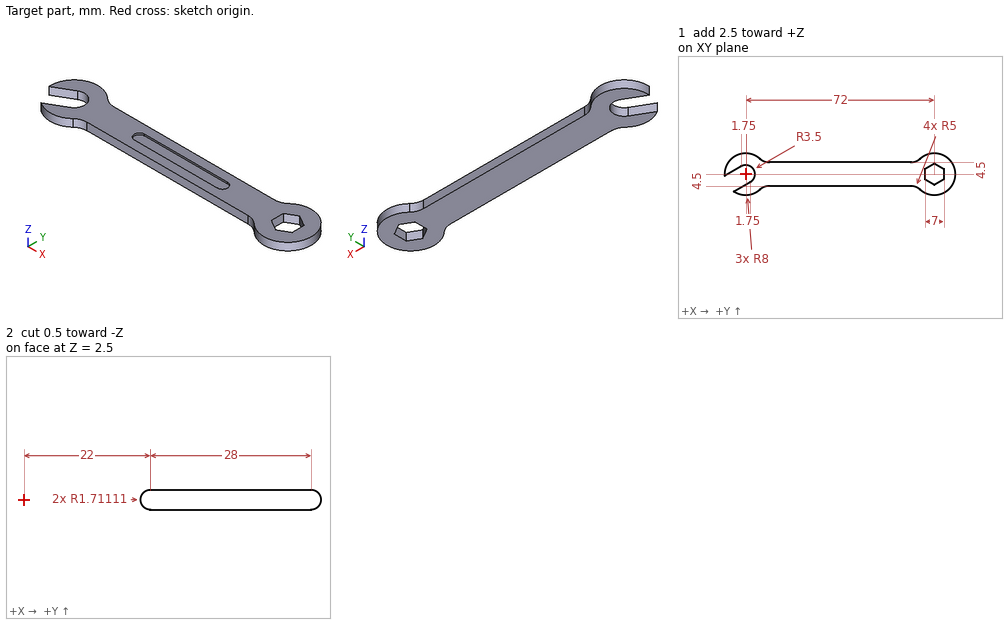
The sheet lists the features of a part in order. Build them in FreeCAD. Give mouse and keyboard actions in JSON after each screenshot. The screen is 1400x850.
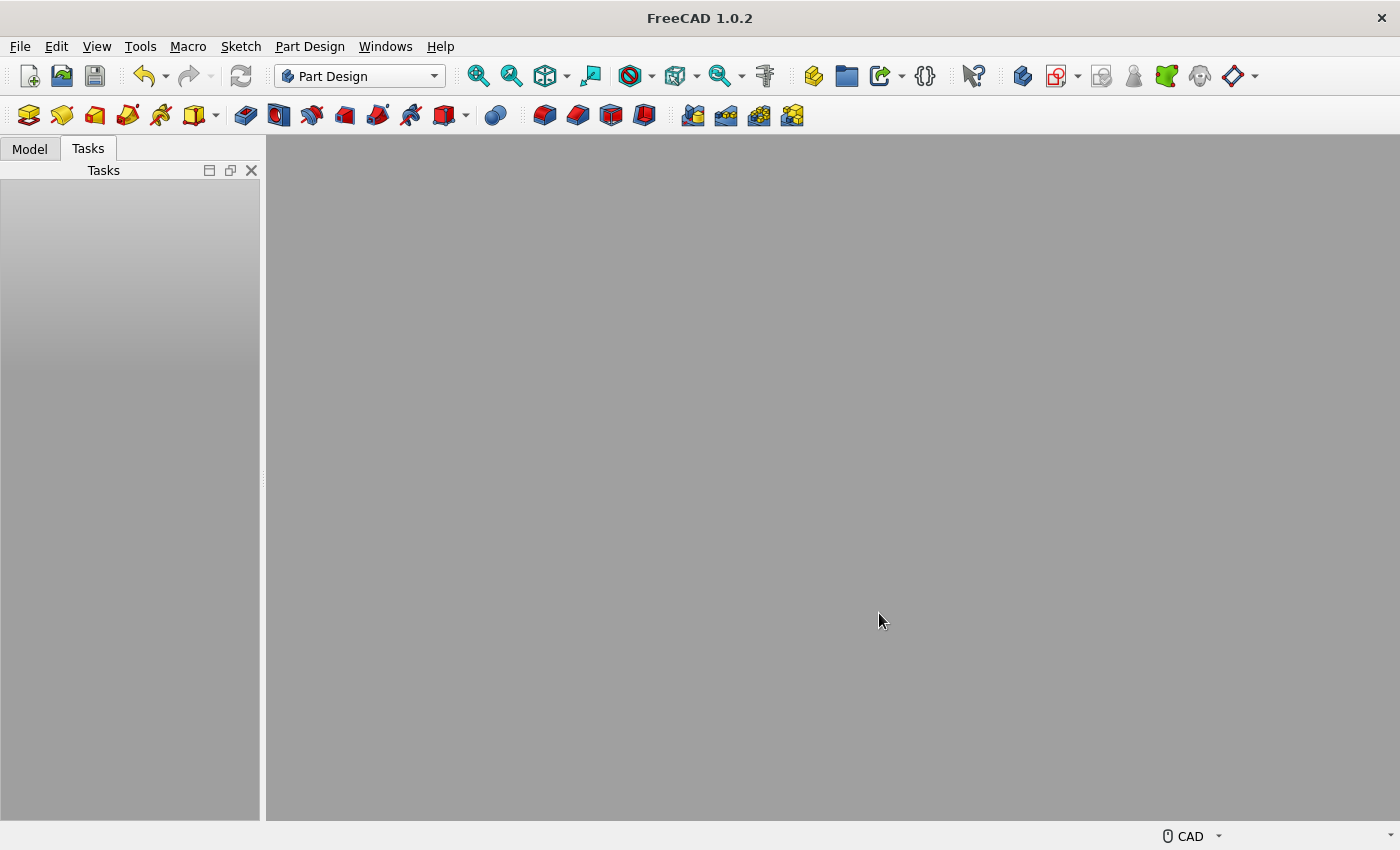
{"action": "left_click", "coordinate": [29, 76]}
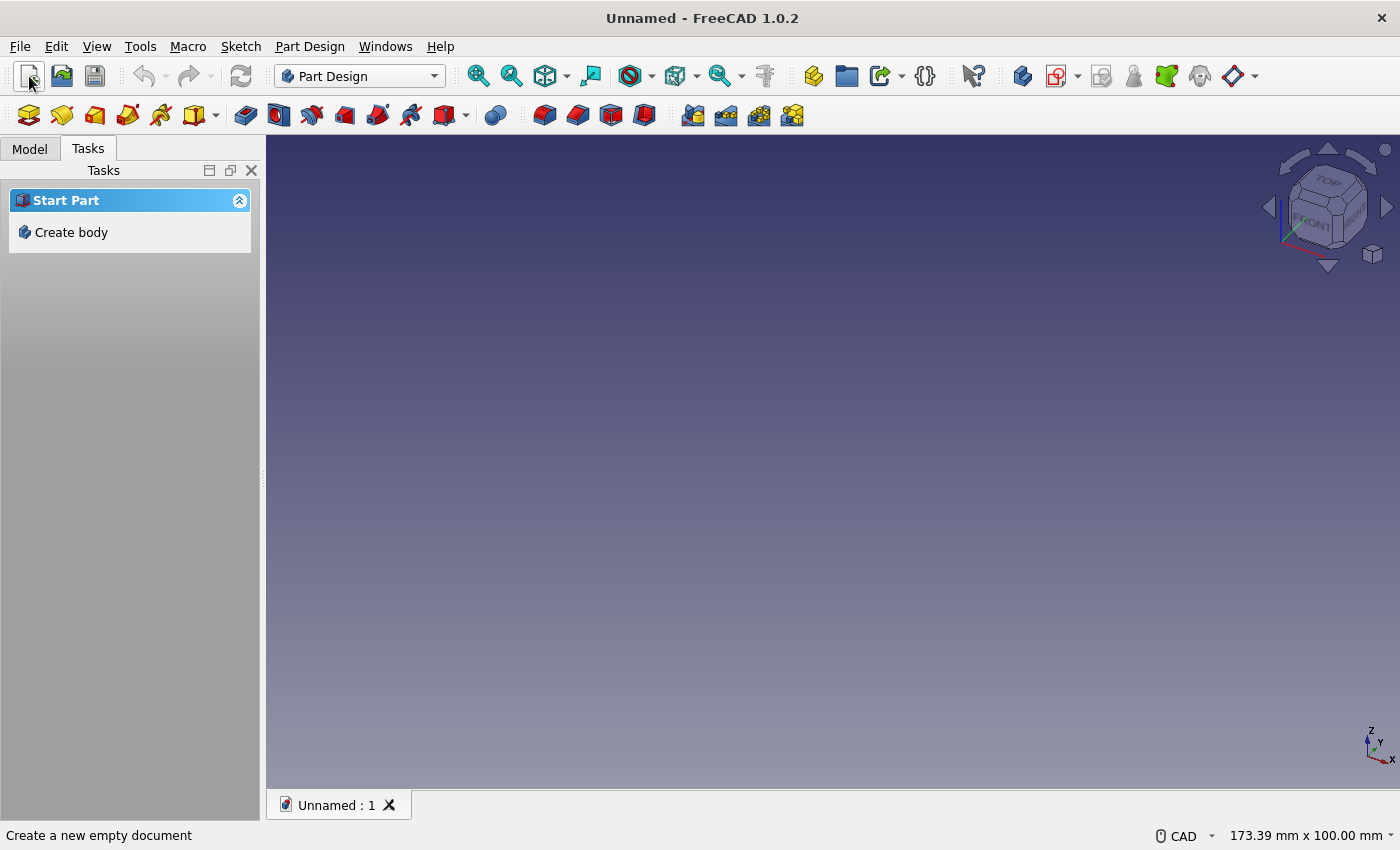
{"action": "left_click", "coordinate": [1056, 76]}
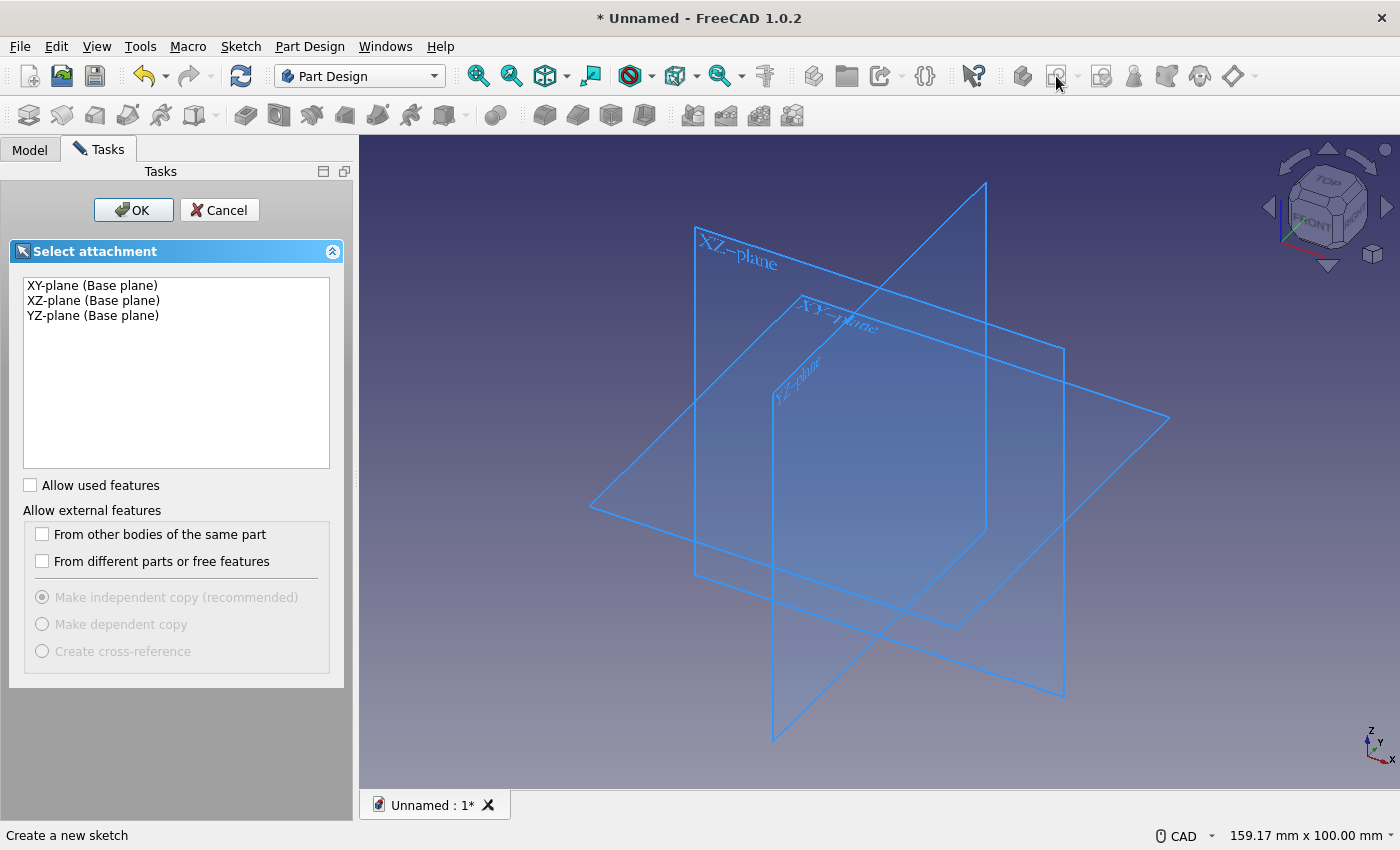
{"action": "left_click", "coordinate": [84, 286]}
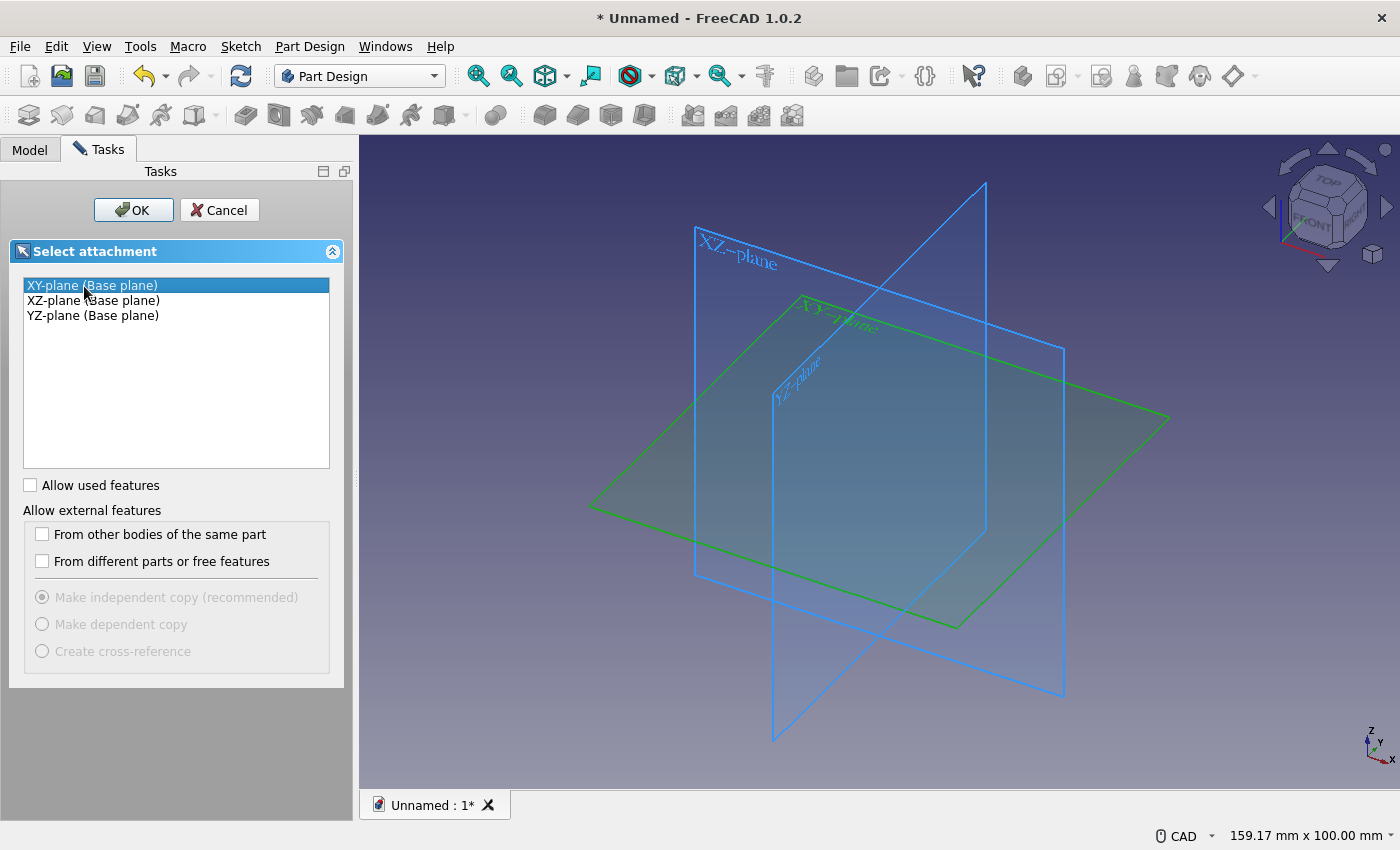
{"action": "left_click", "coordinate": [134, 210]}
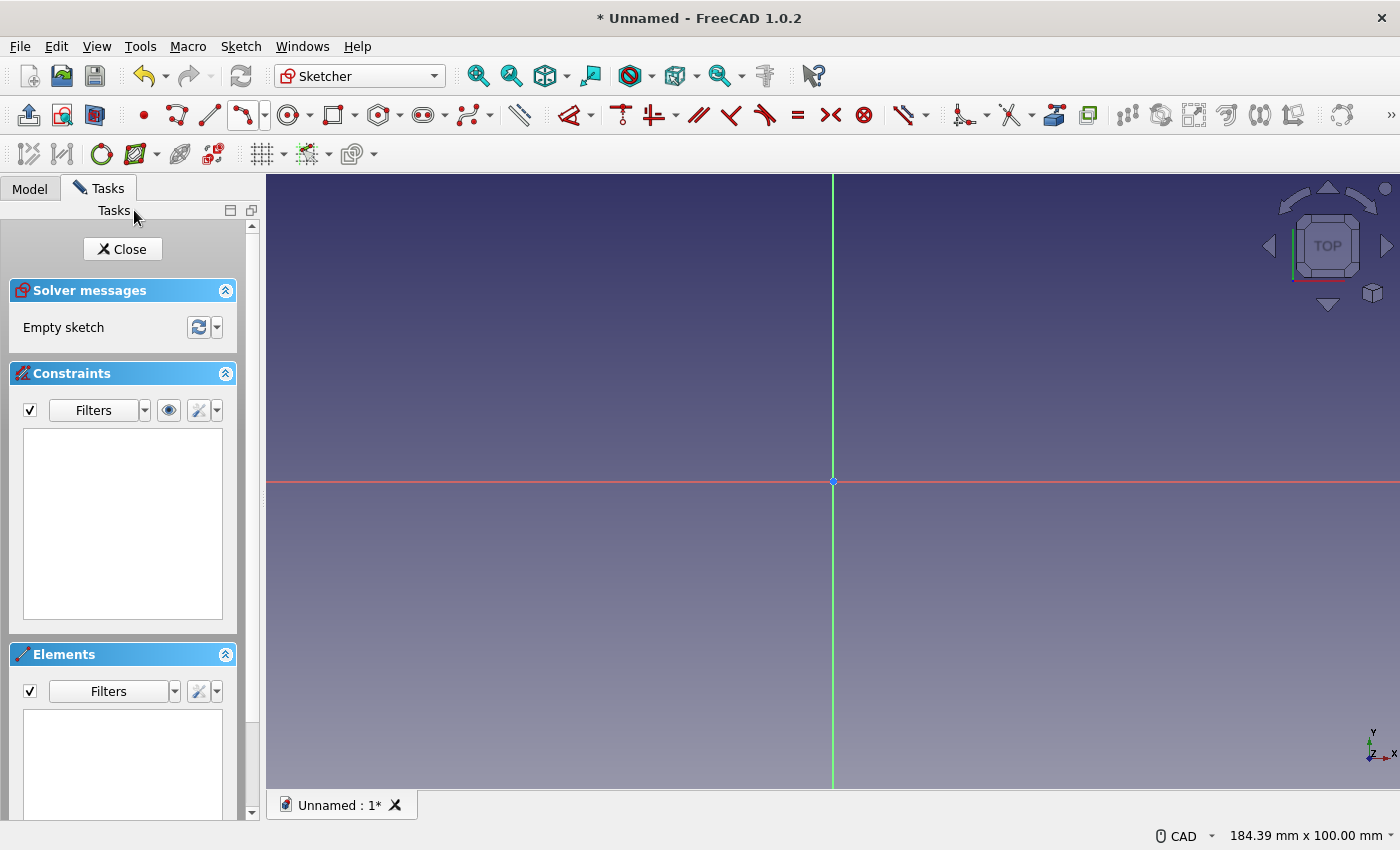
{"action": "scroll", "coordinate": [294, 471], "scroll_direction": "down", "scroll_amount": 1}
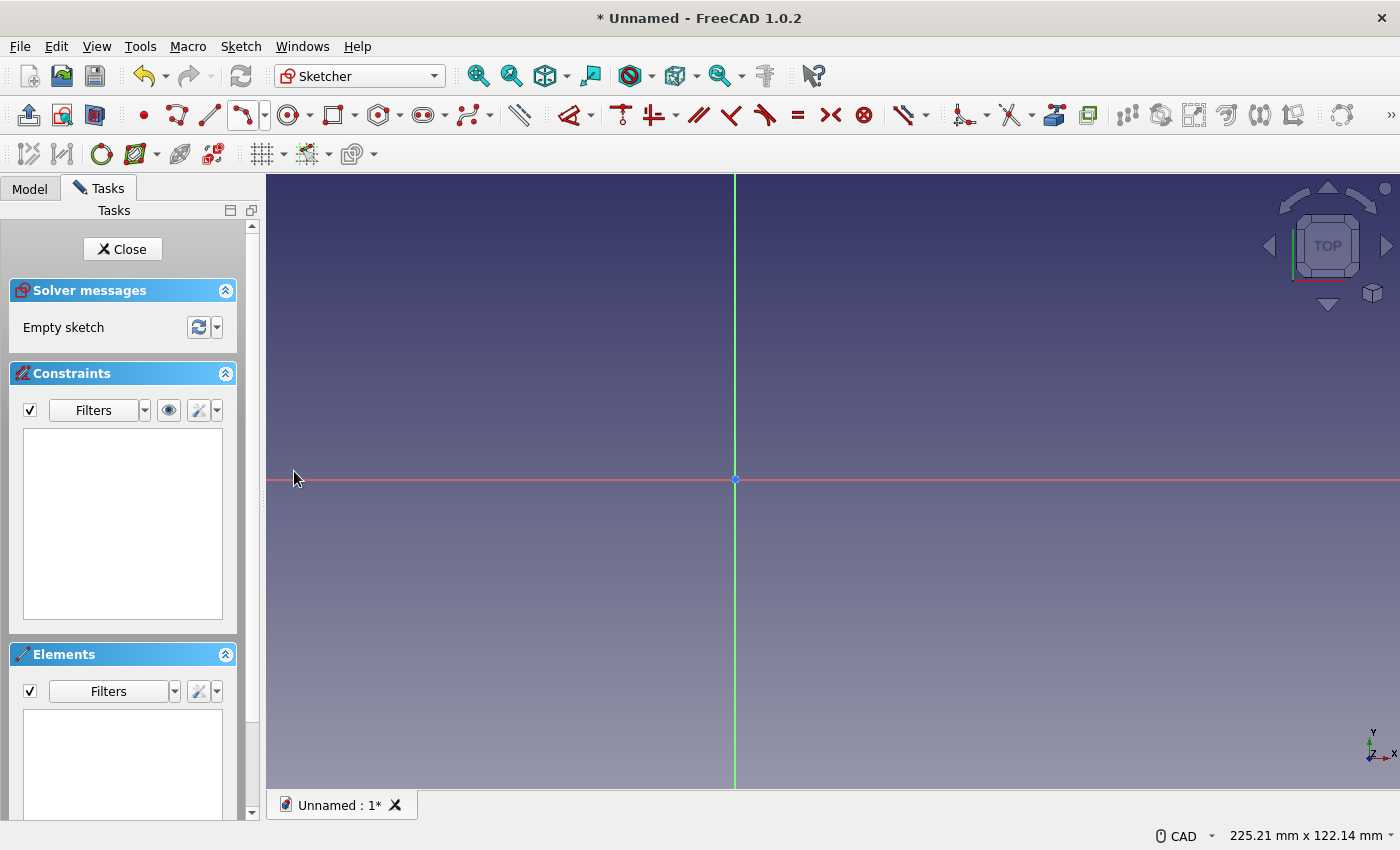
{"action": "scroll", "coordinate": [1226, 482], "scroll_direction": "up", "scroll_amount": 2}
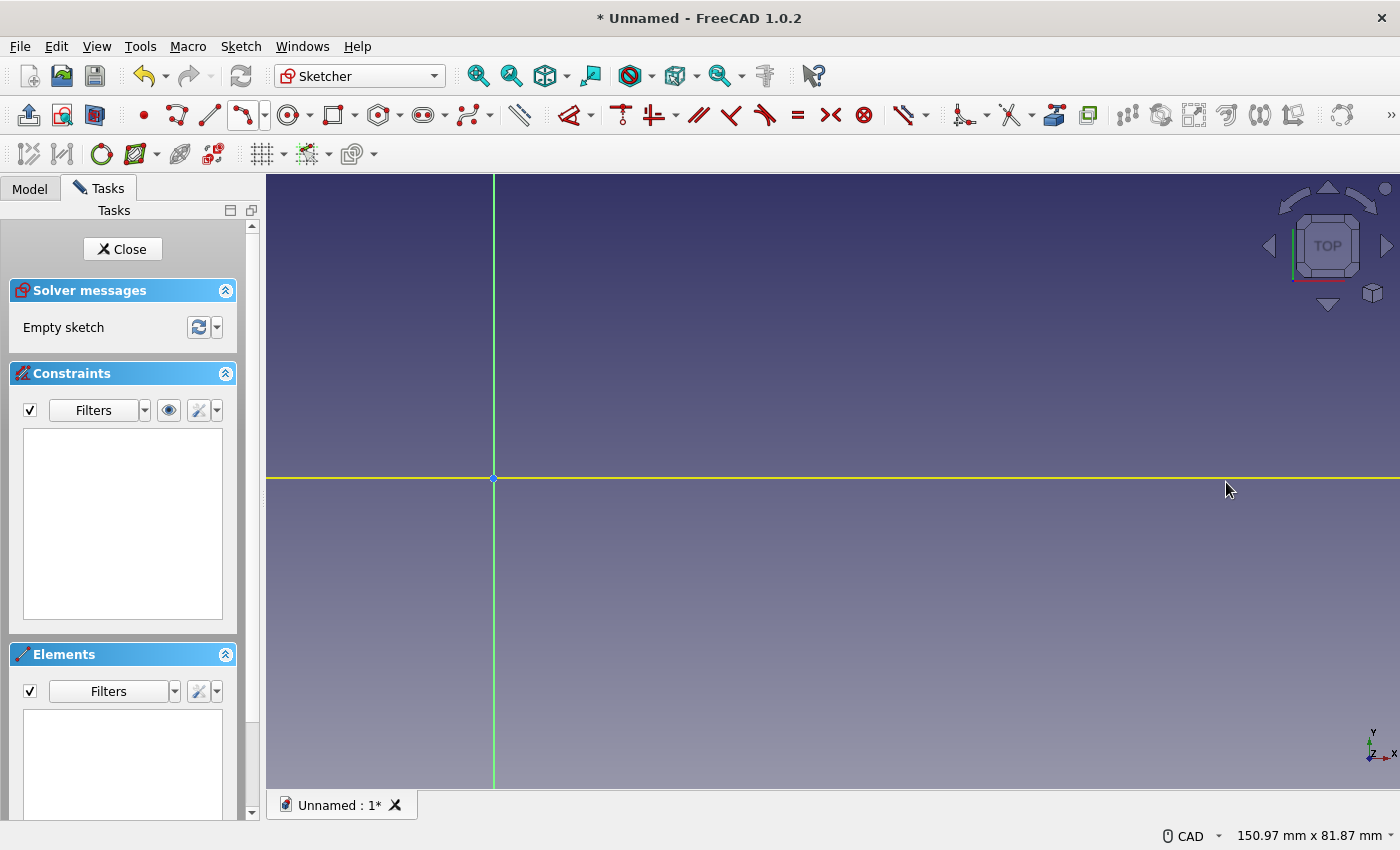
{"action": "left_click", "coordinate": [210, 116]}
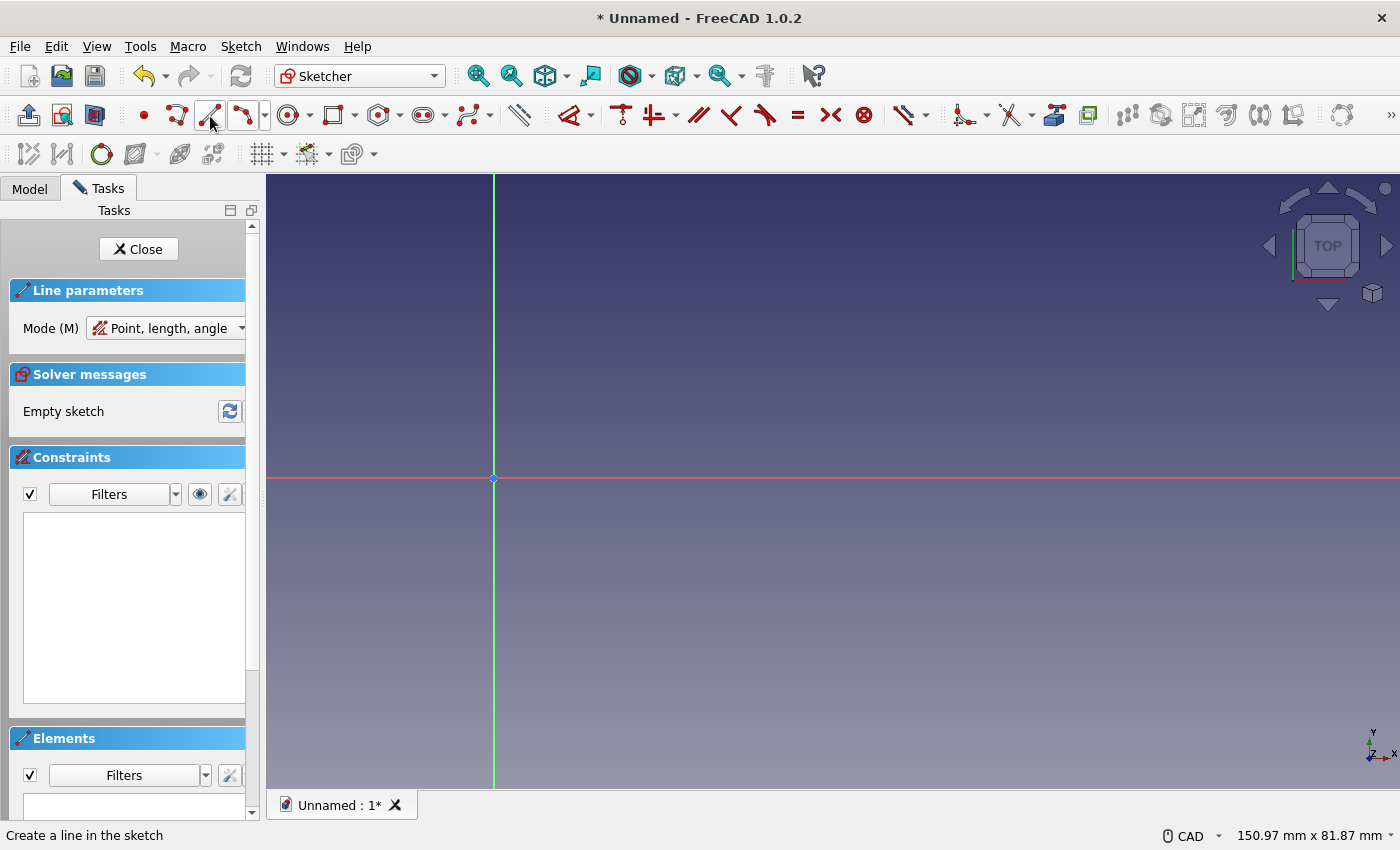
{"action": "left_click", "coordinate": [560, 512]}
{"action": "left_click", "coordinate": [968, 512]}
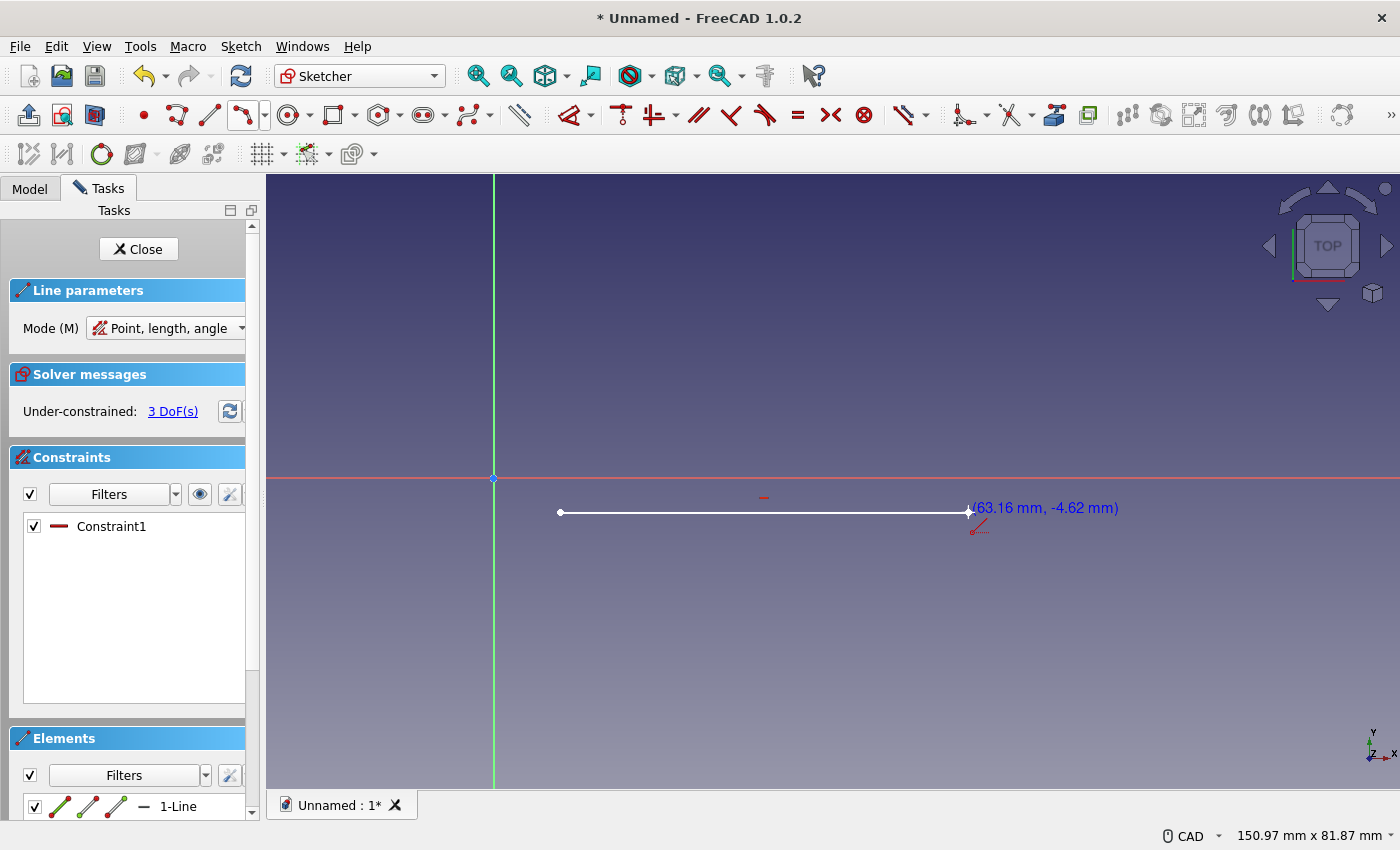
{"action": "left_click", "coordinate": [968, 444]}
{"action": "left_click", "coordinate": [560, 444]}